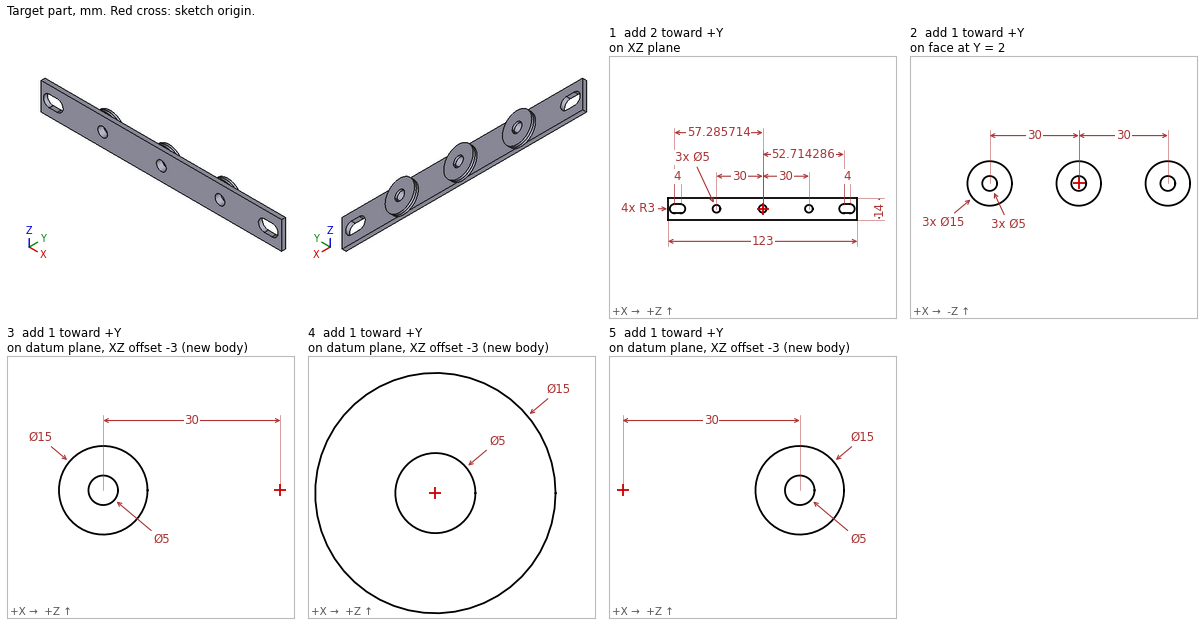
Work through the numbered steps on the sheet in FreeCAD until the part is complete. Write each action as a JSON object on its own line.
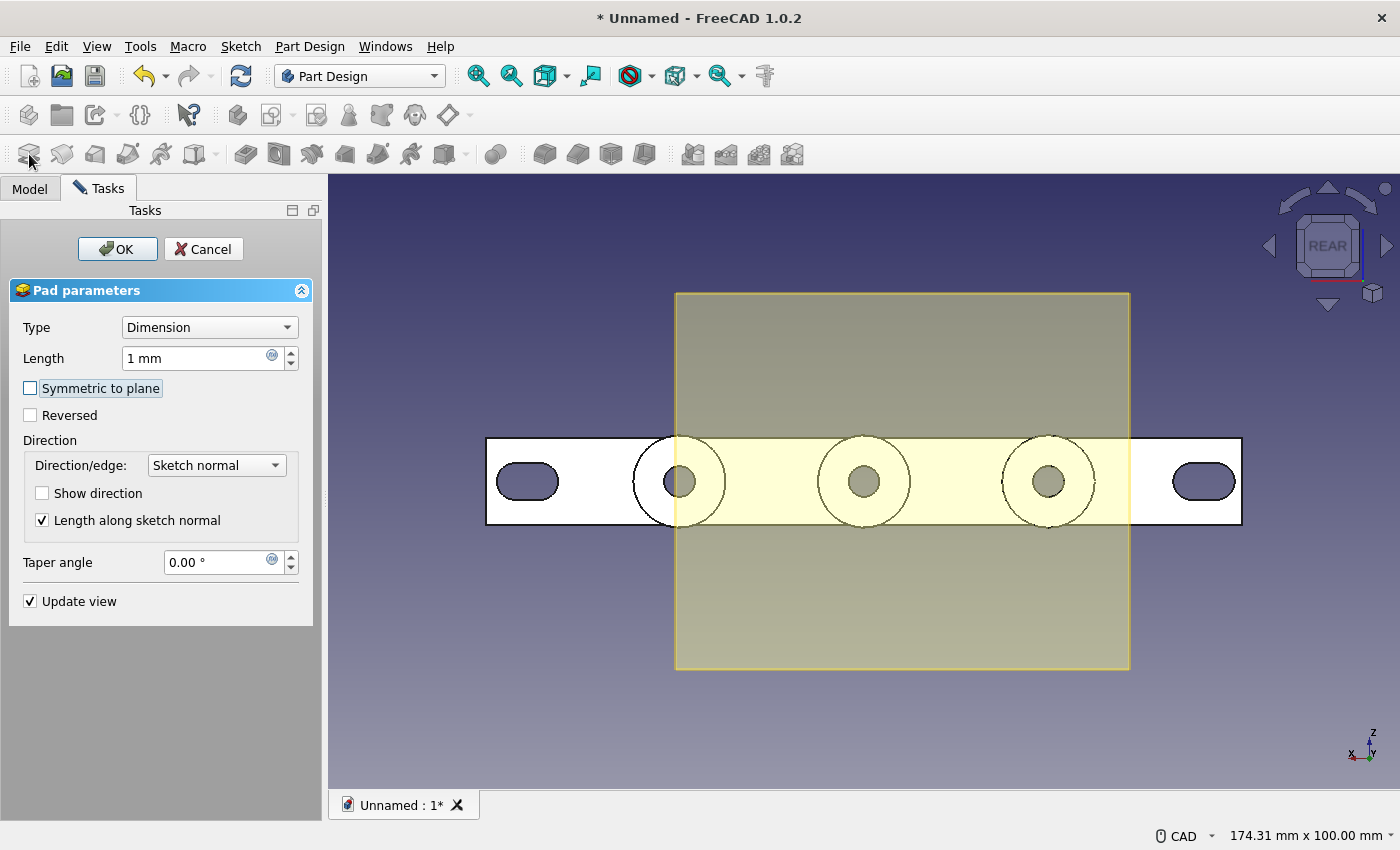
{"action": "left_click", "coordinate": [31, 415]}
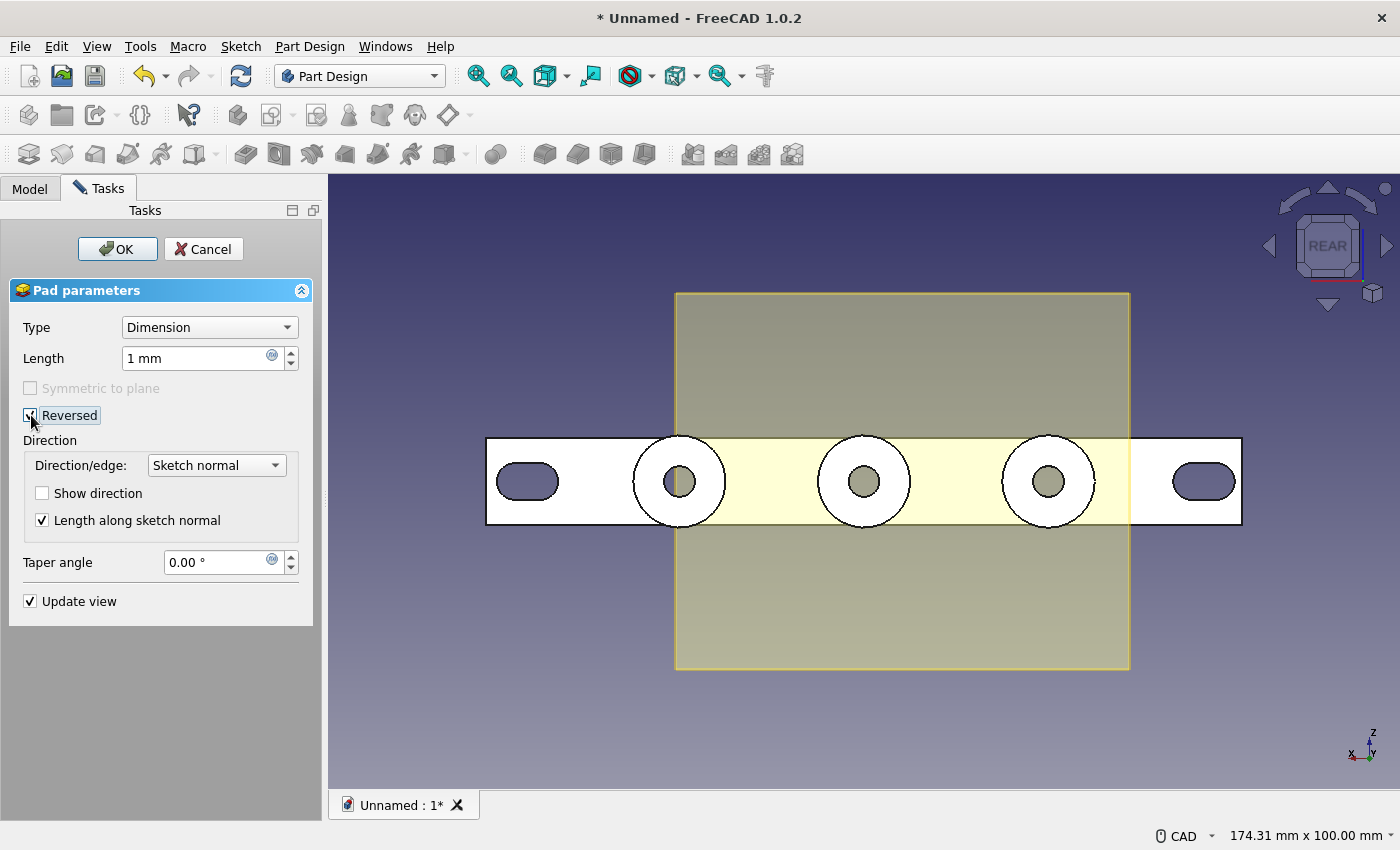
{"action": "left_click", "coordinate": [118, 249]}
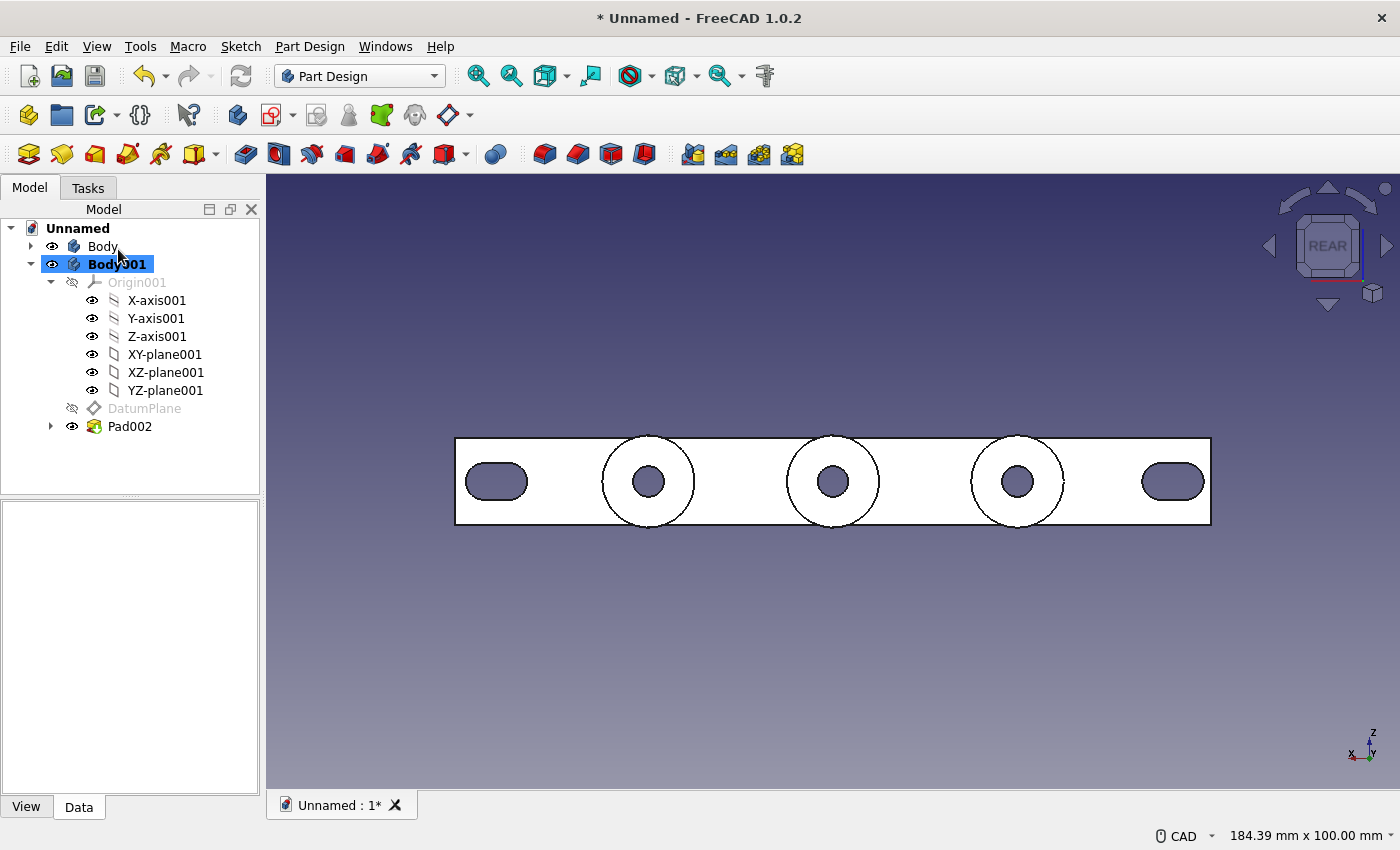
{"action": "left_click", "coordinate": [479, 76]}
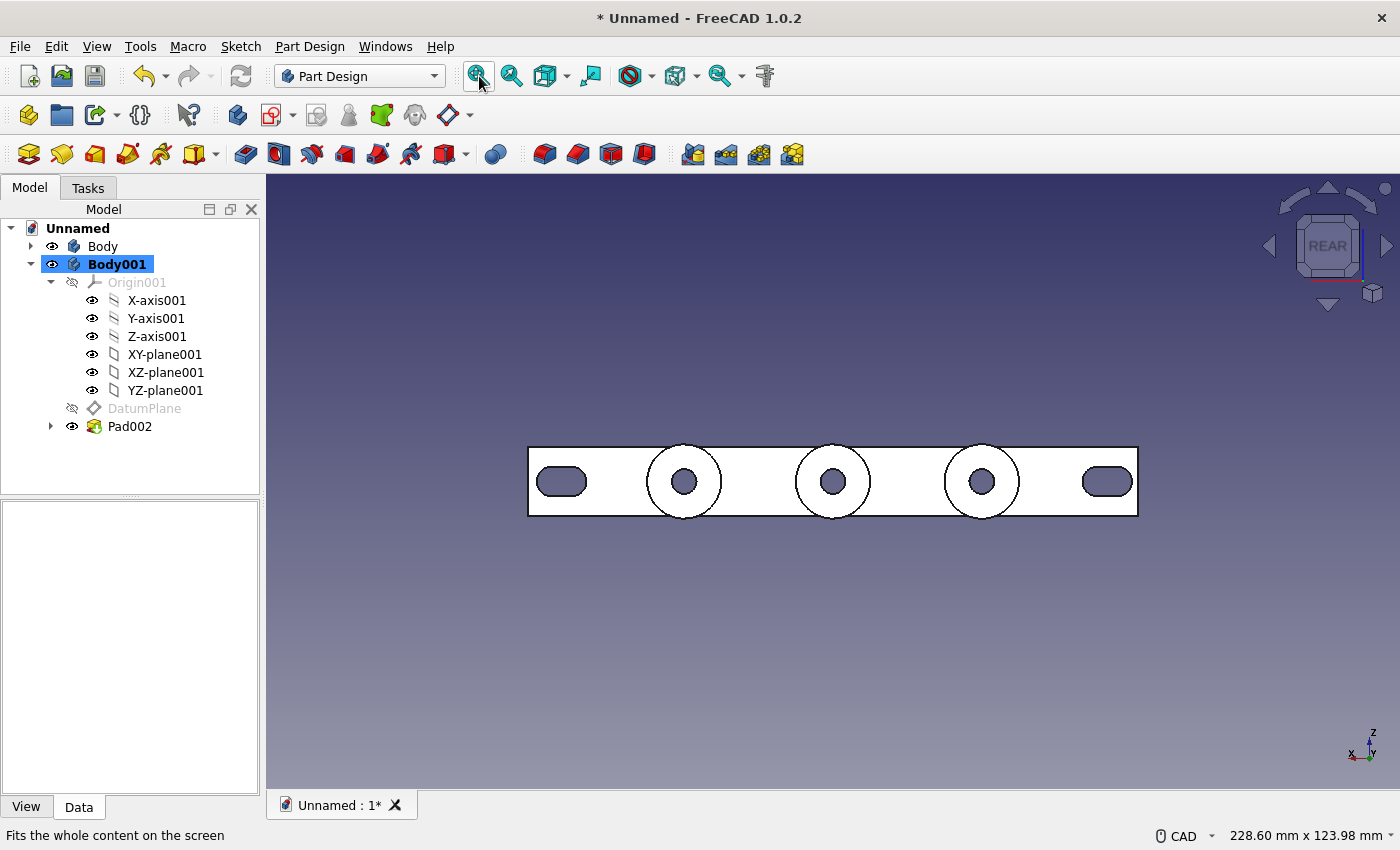
{"action": "left_click", "coordinate": [238, 116]}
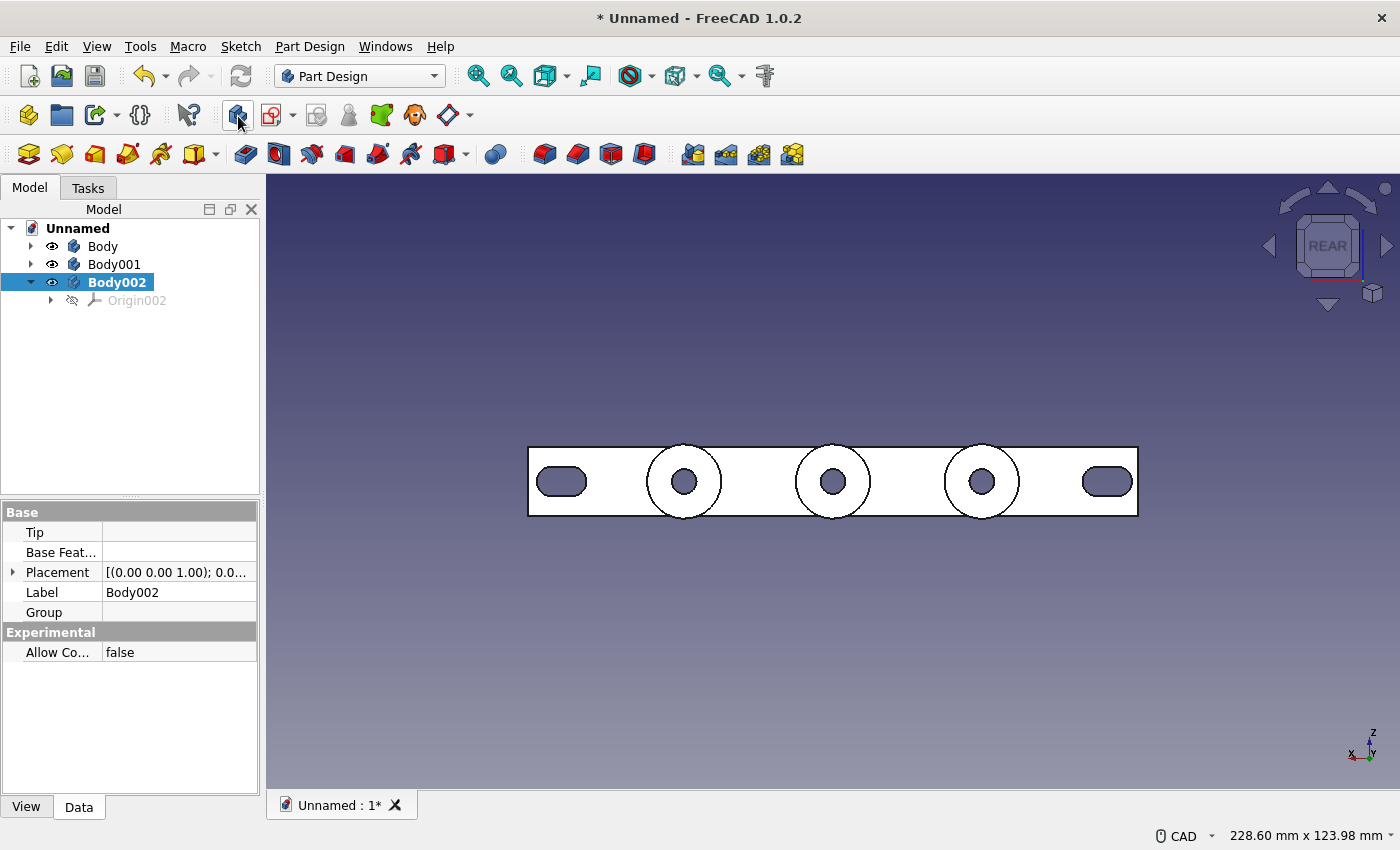
{"action": "left_click", "coordinate": [51, 300]}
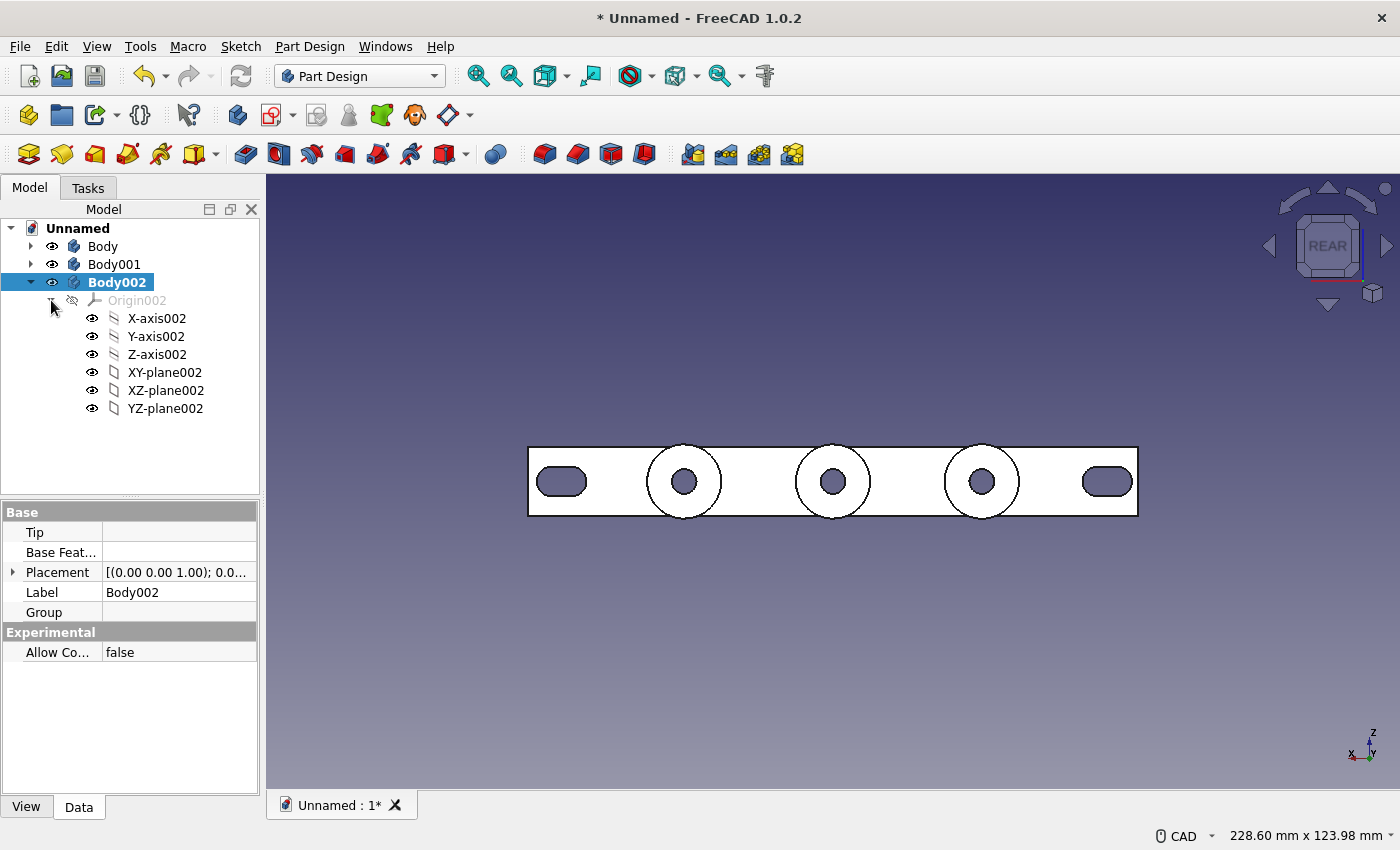
{"action": "left_click", "coordinate": [137, 390]}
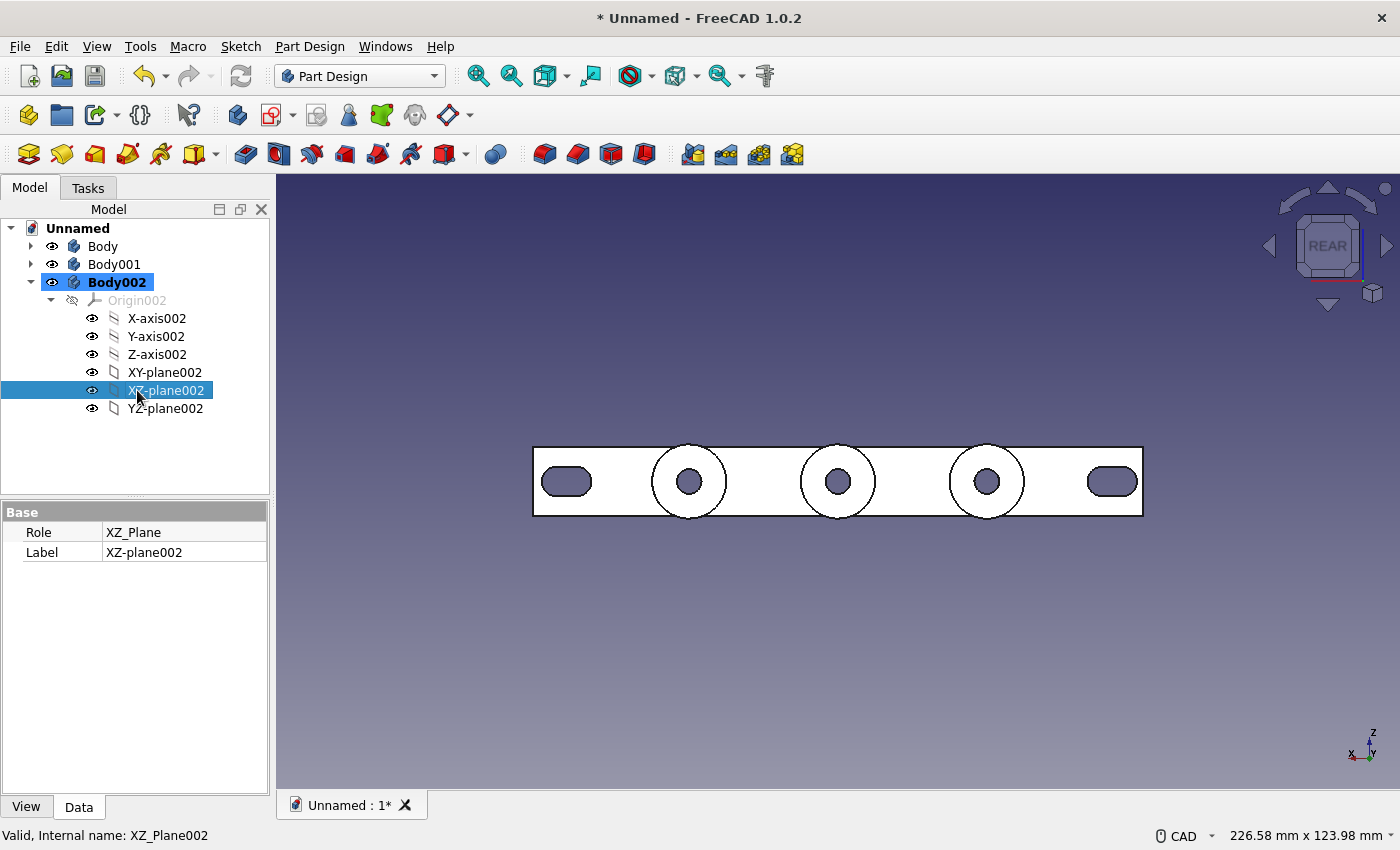
{"action": "left_click", "coordinate": [448, 116]}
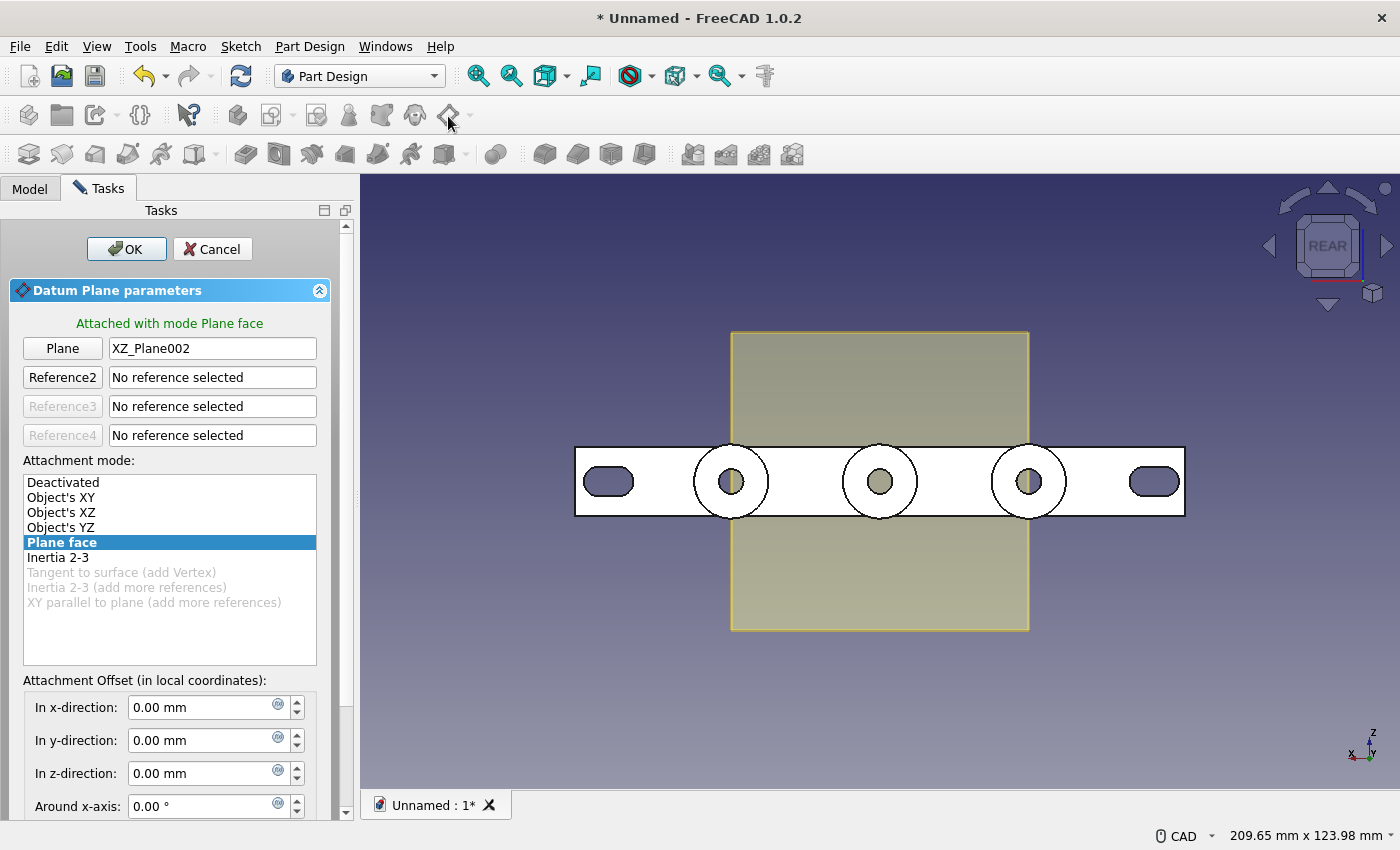
{"action": "triple_click", "coordinate": [210, 774]}